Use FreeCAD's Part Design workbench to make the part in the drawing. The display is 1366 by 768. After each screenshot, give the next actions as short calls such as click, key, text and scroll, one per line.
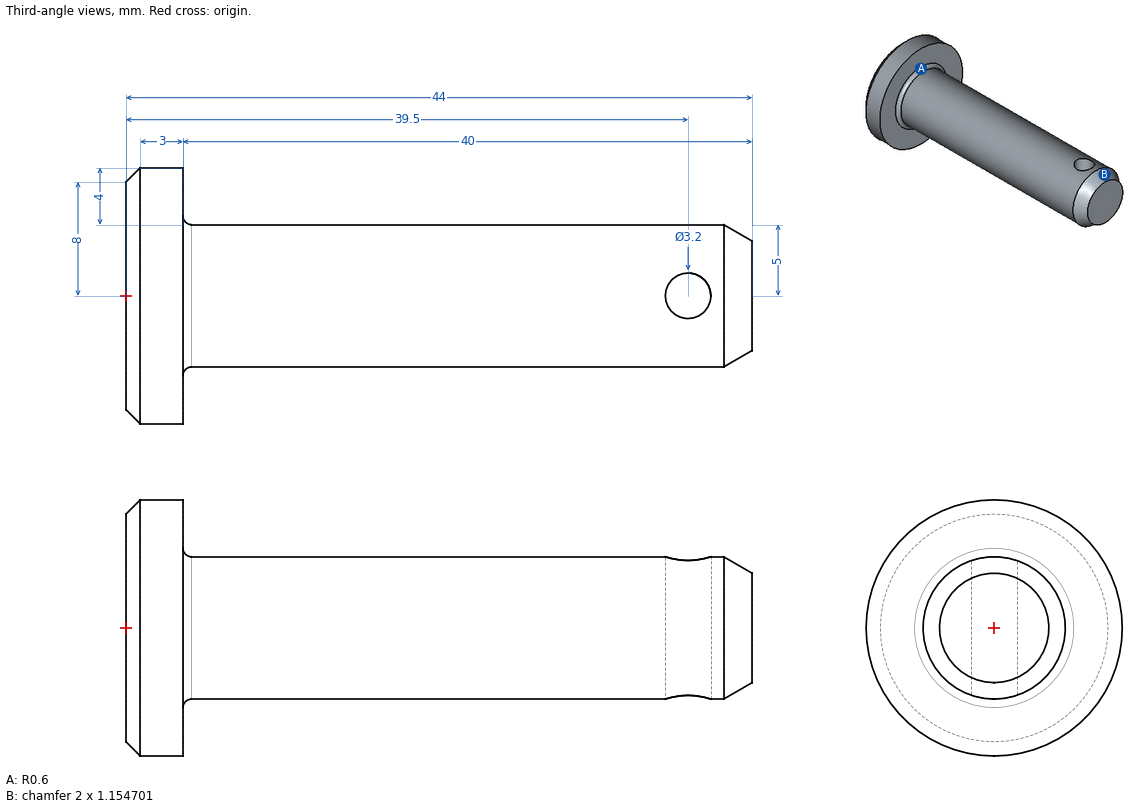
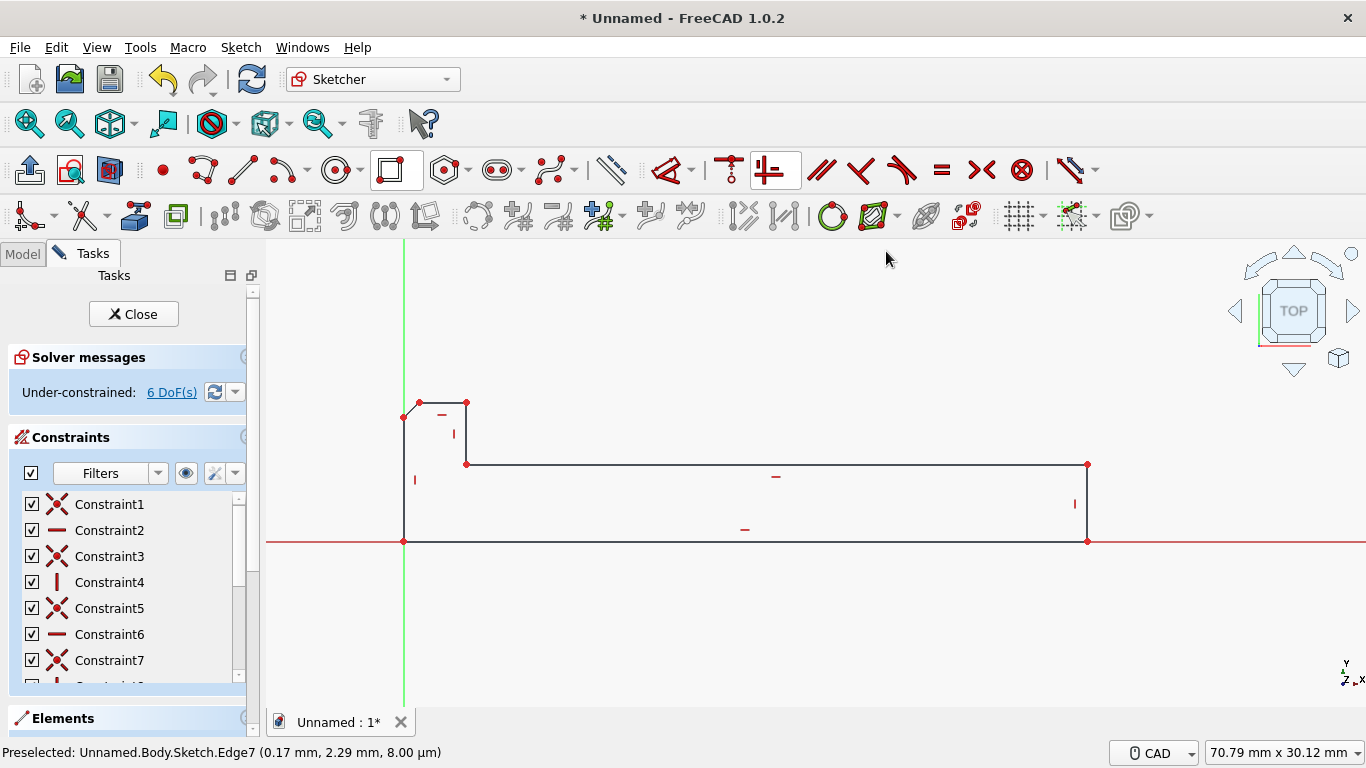
click(1087, 519)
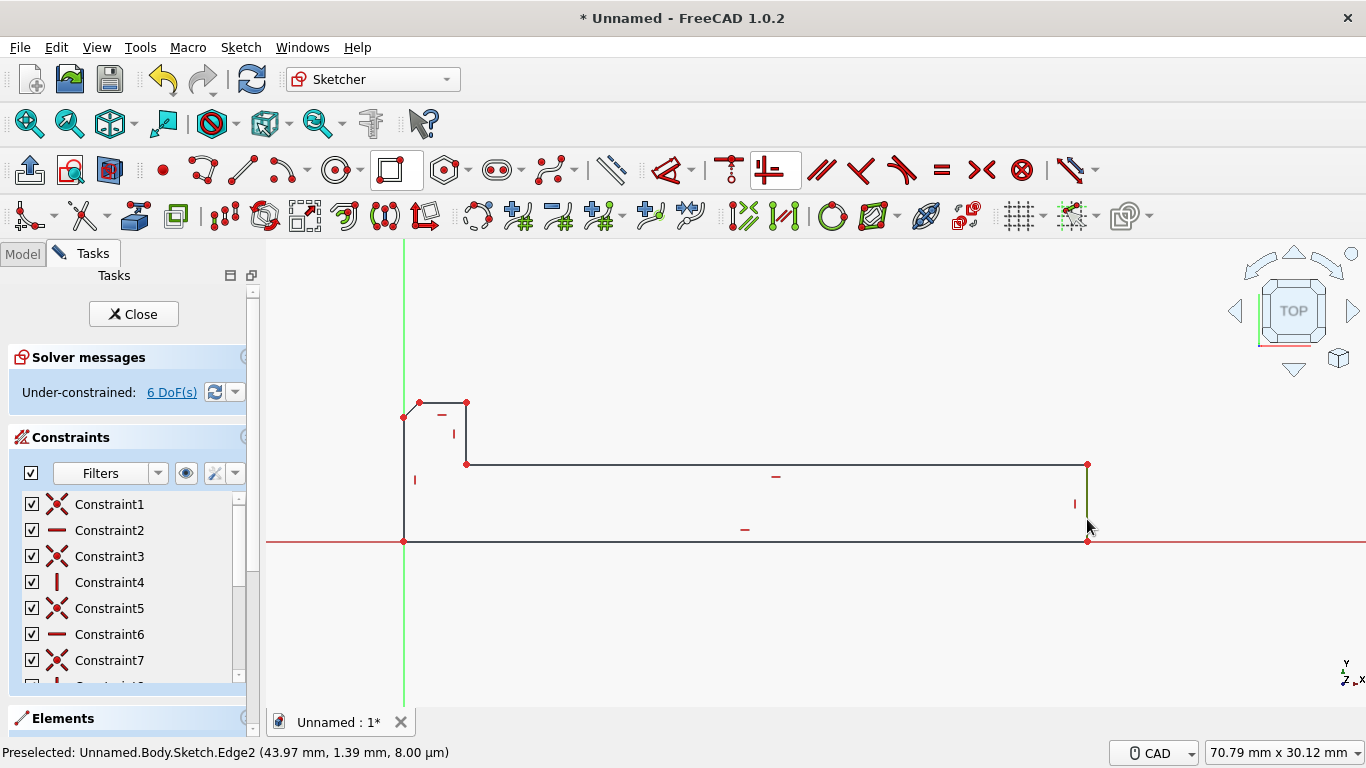
key(i)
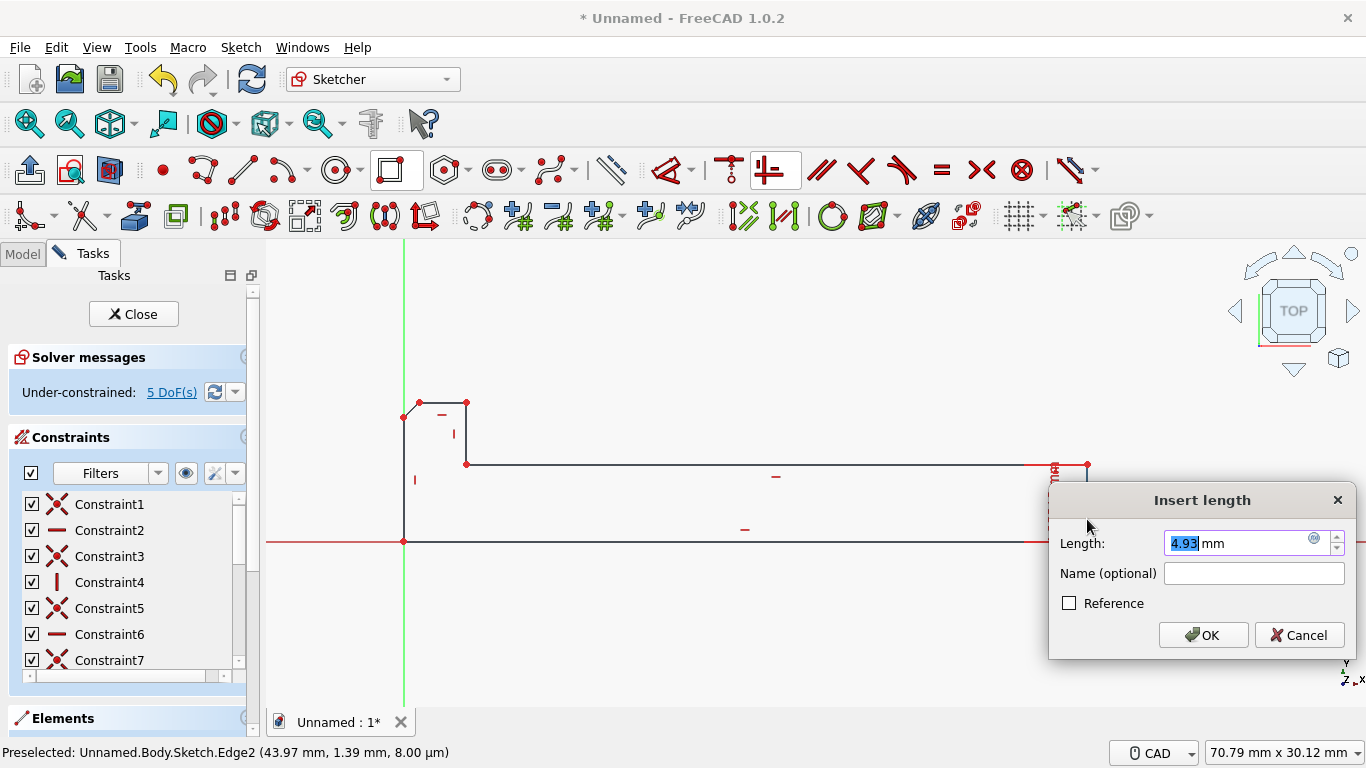
text(5)
key(Return)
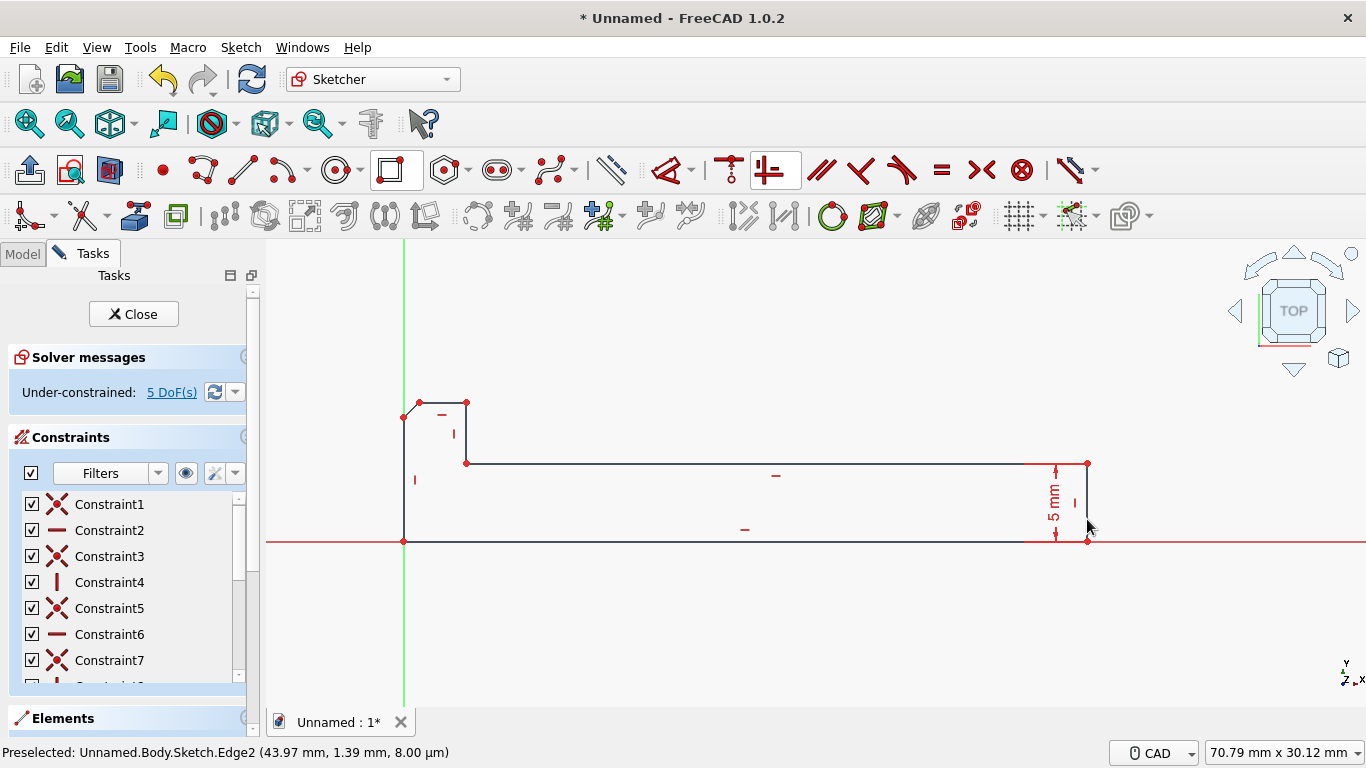
click(466, 446)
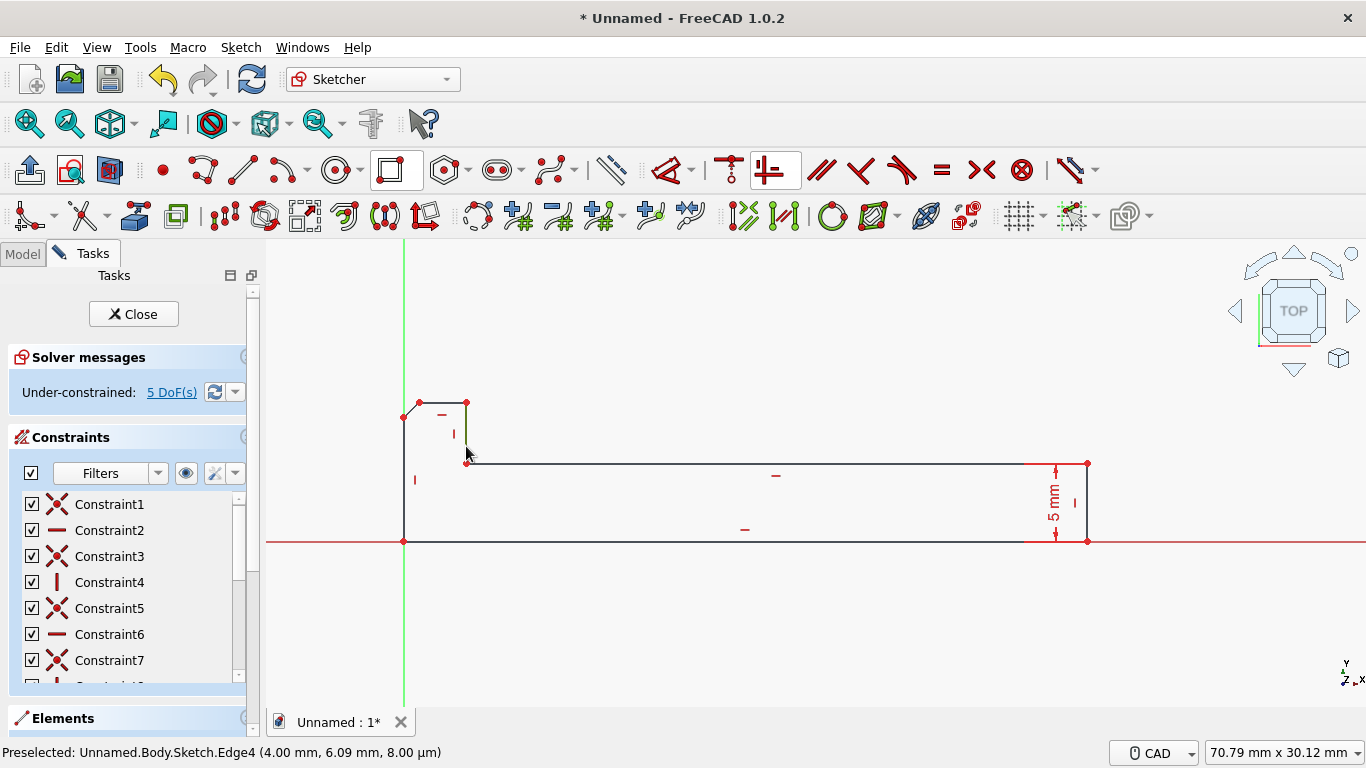
key(i)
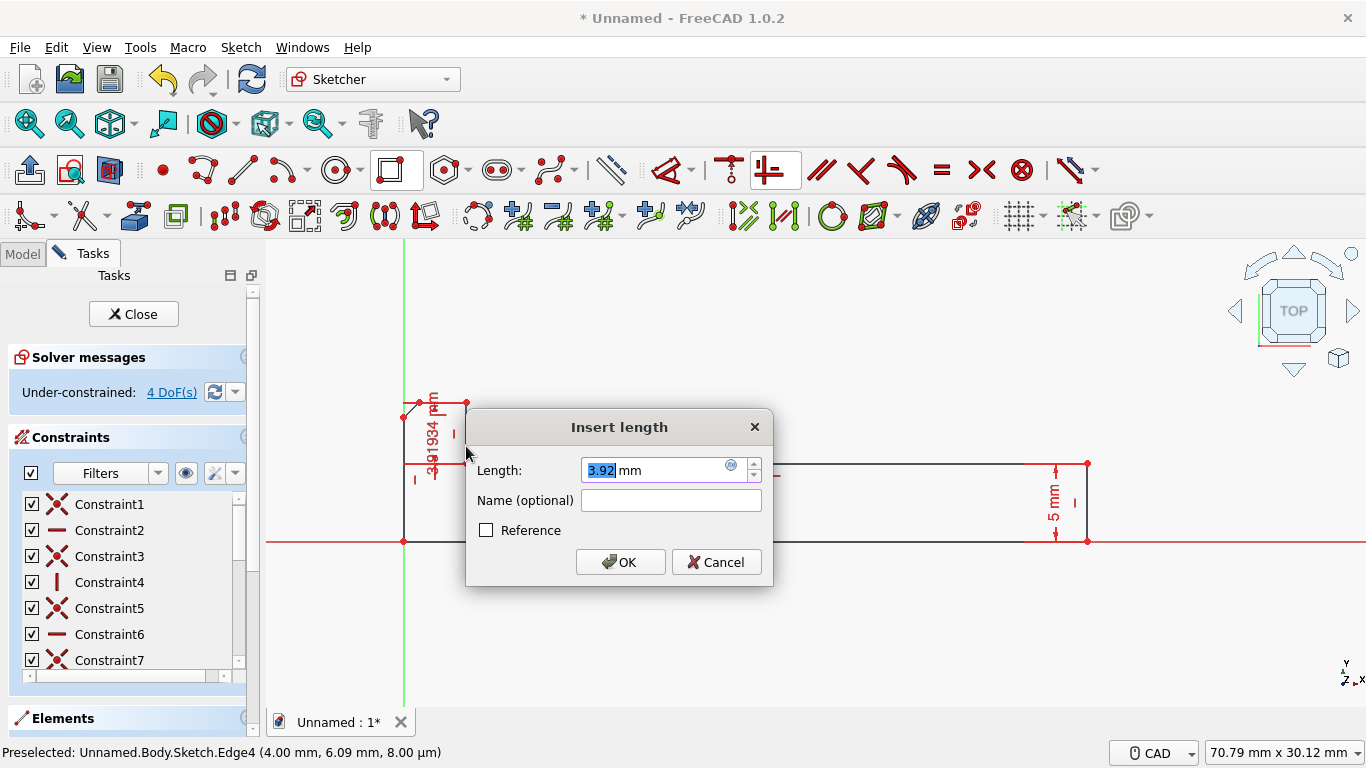
text(4)
key(Return)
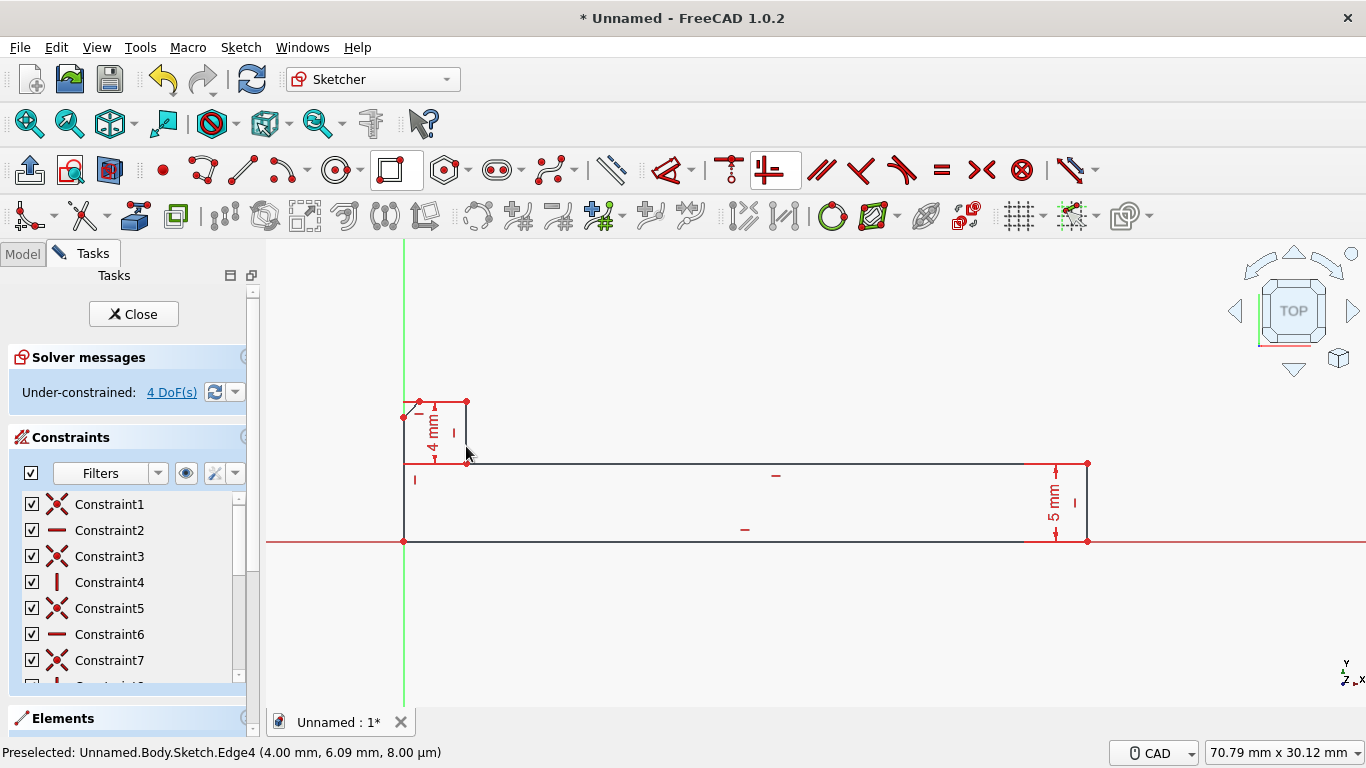
click(452, 402)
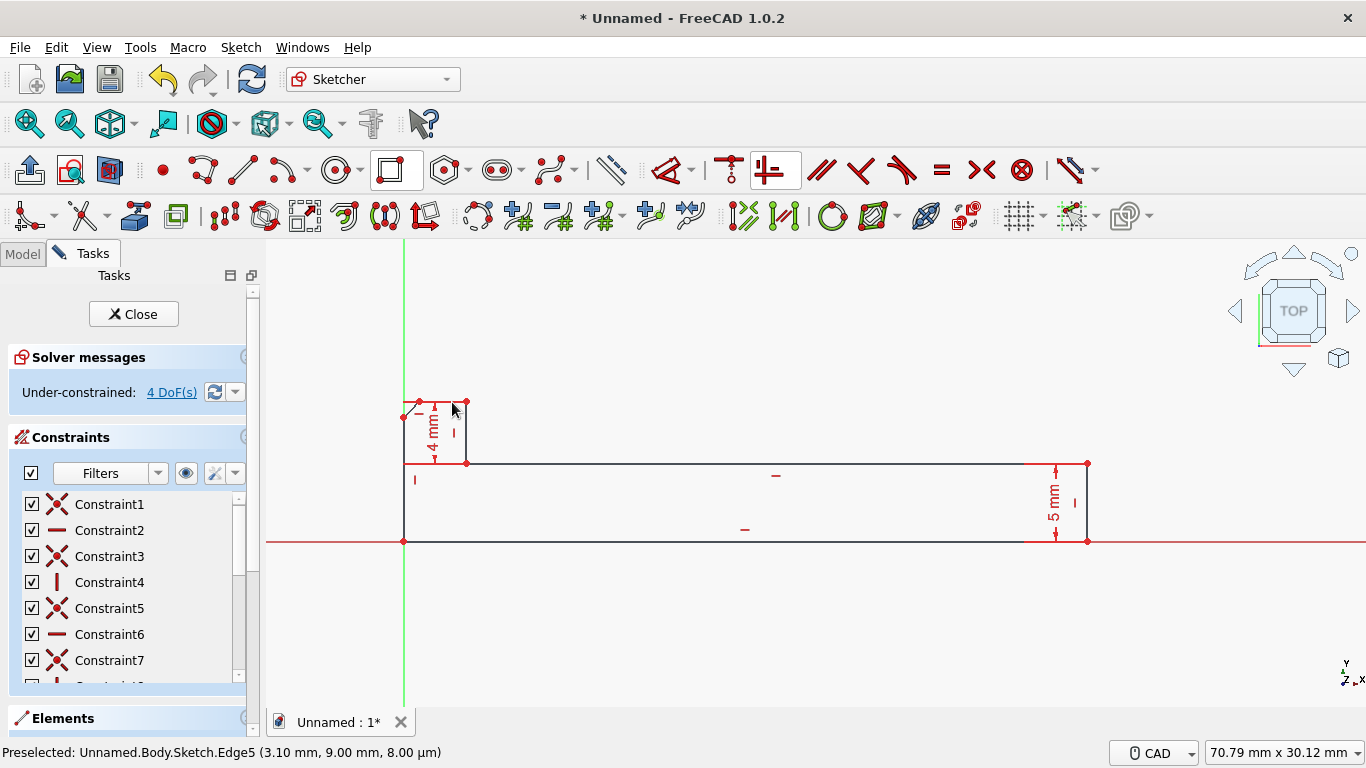
click(694, 170)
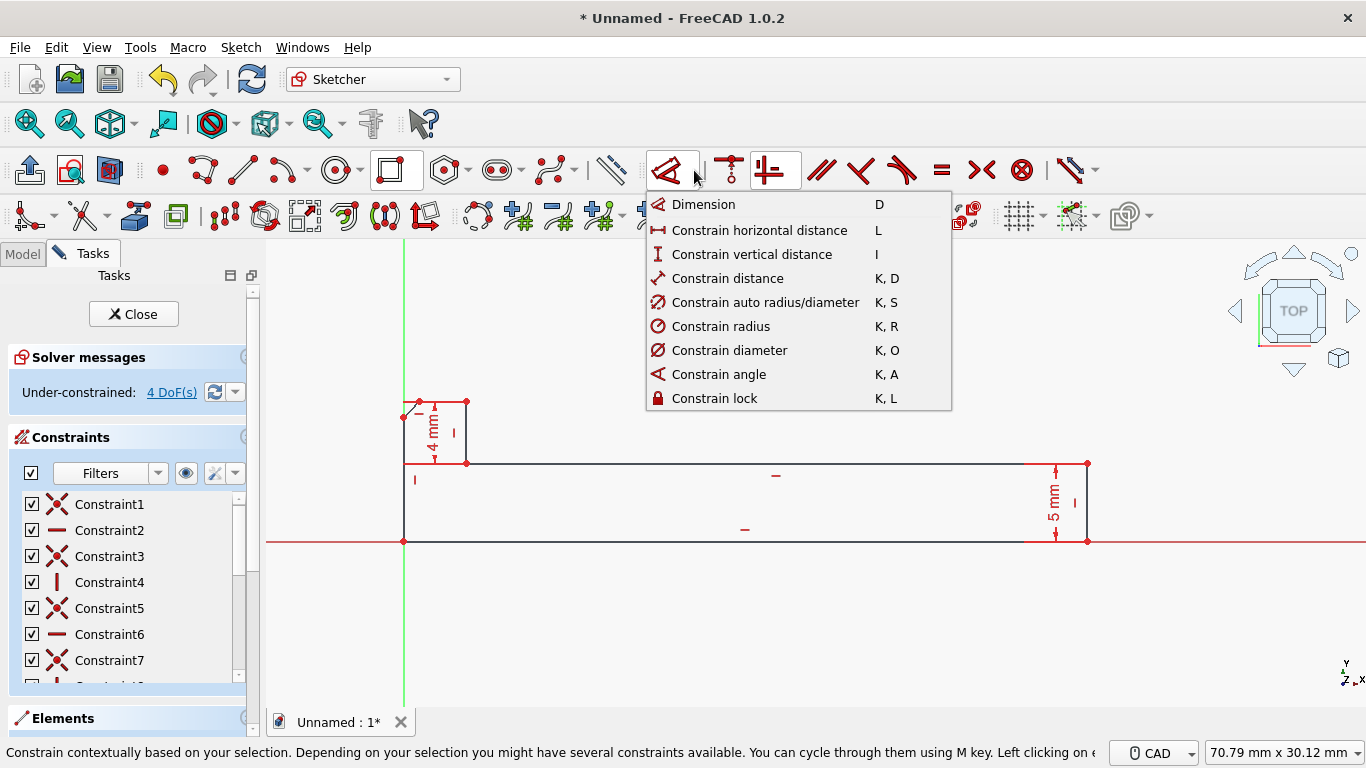
click(799, 230)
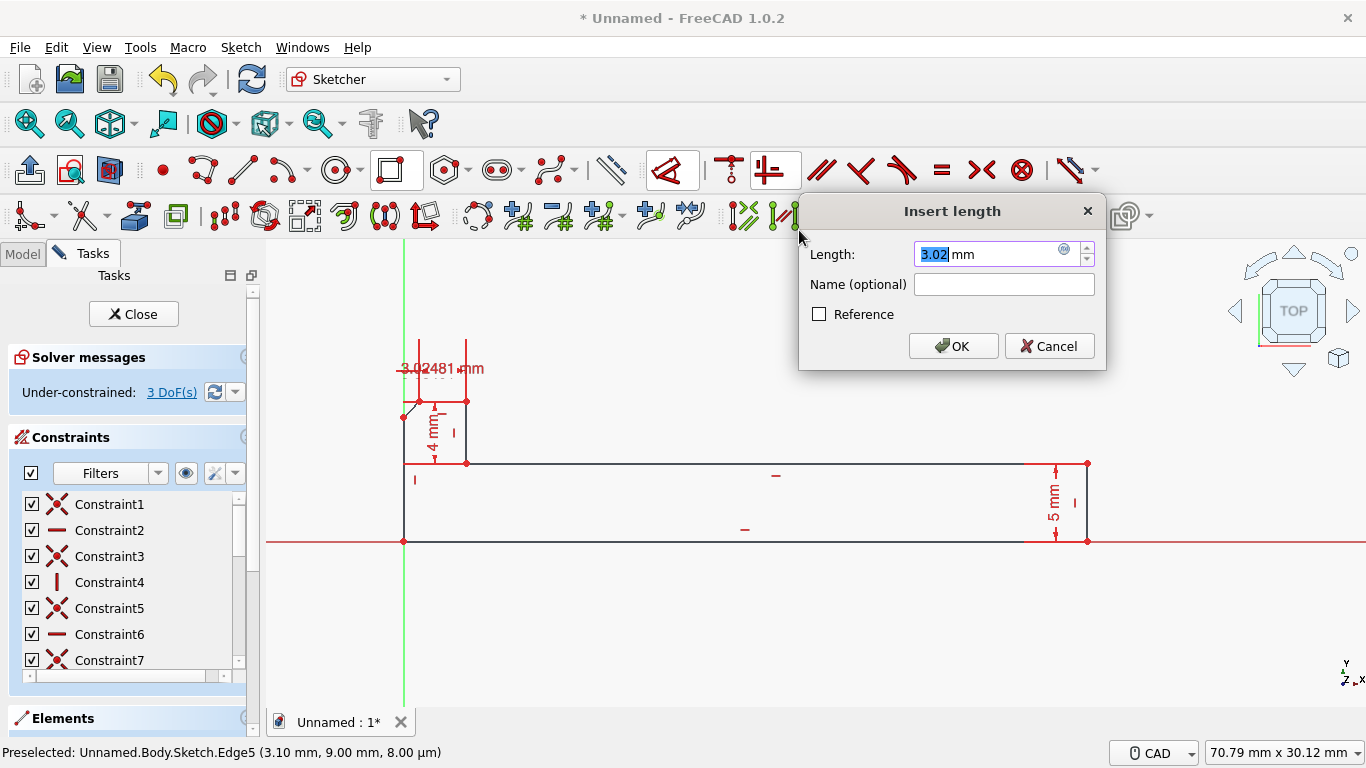
text(3)
key(Return)